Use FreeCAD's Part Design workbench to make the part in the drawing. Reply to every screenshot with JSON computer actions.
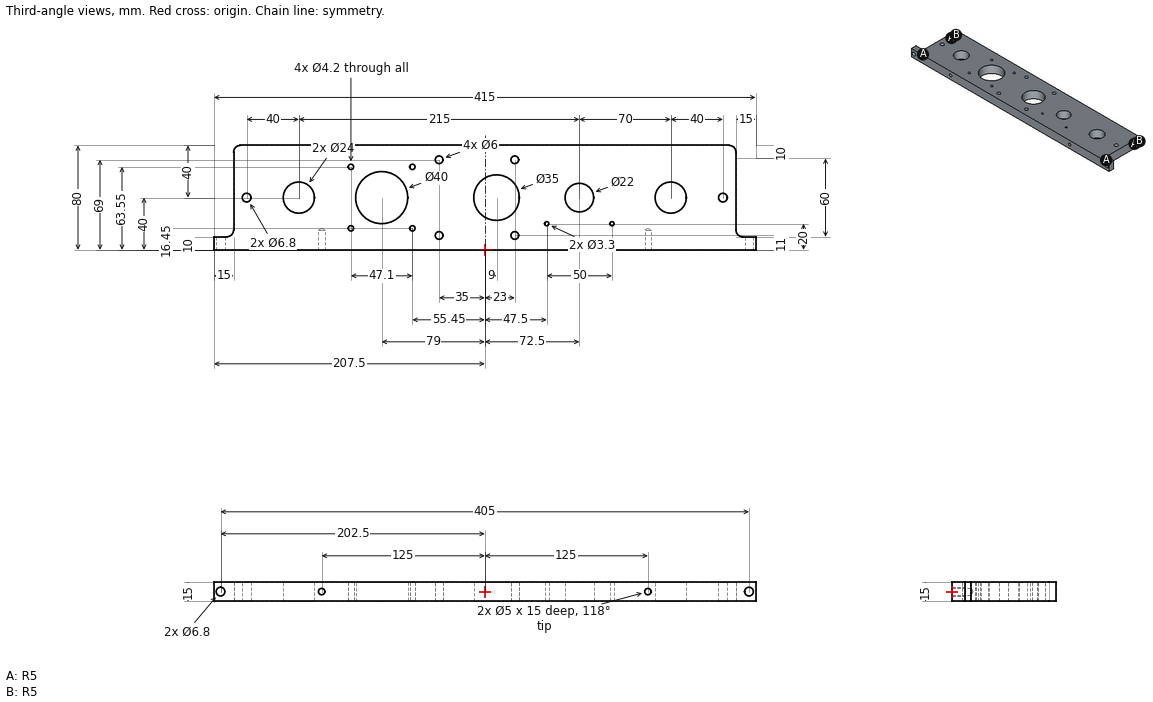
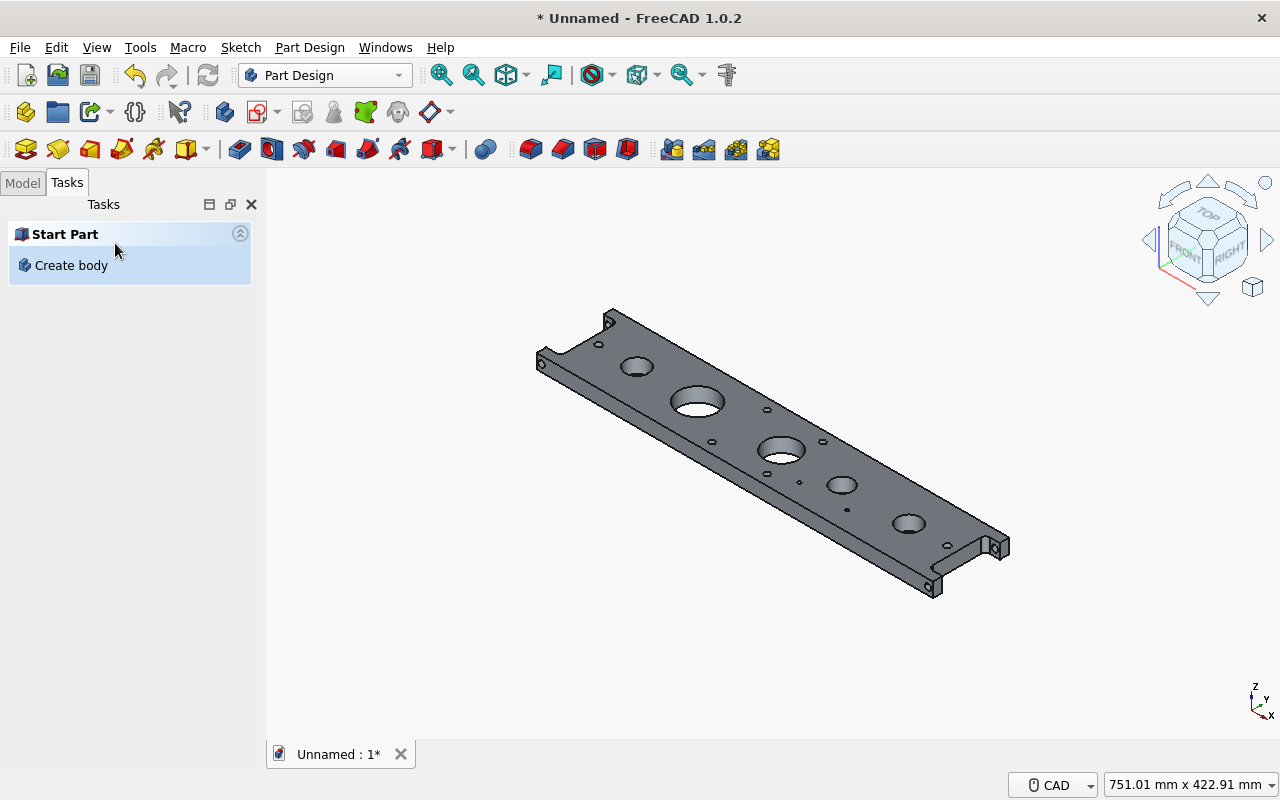
{"action": "left_click", "coordinate": [908, 497]}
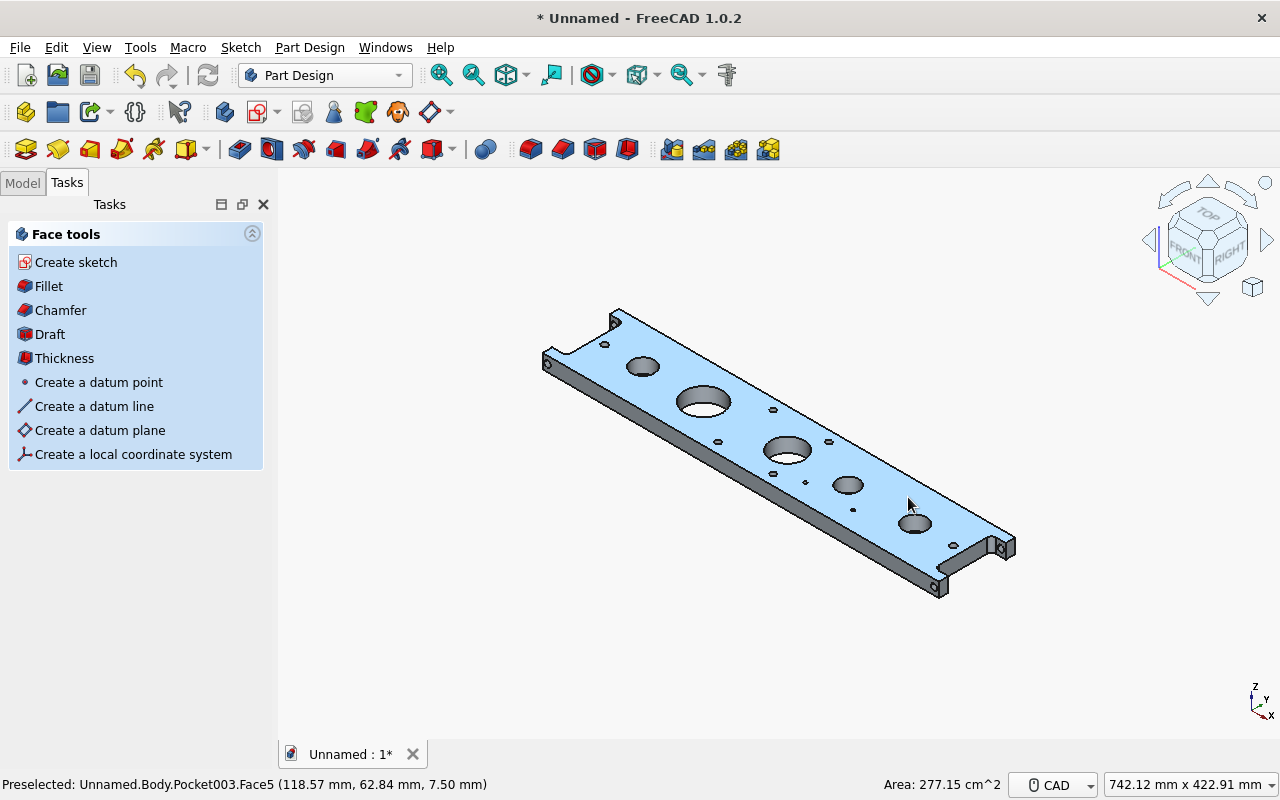
{"action": "left_click", "coordinate": [258, 112]}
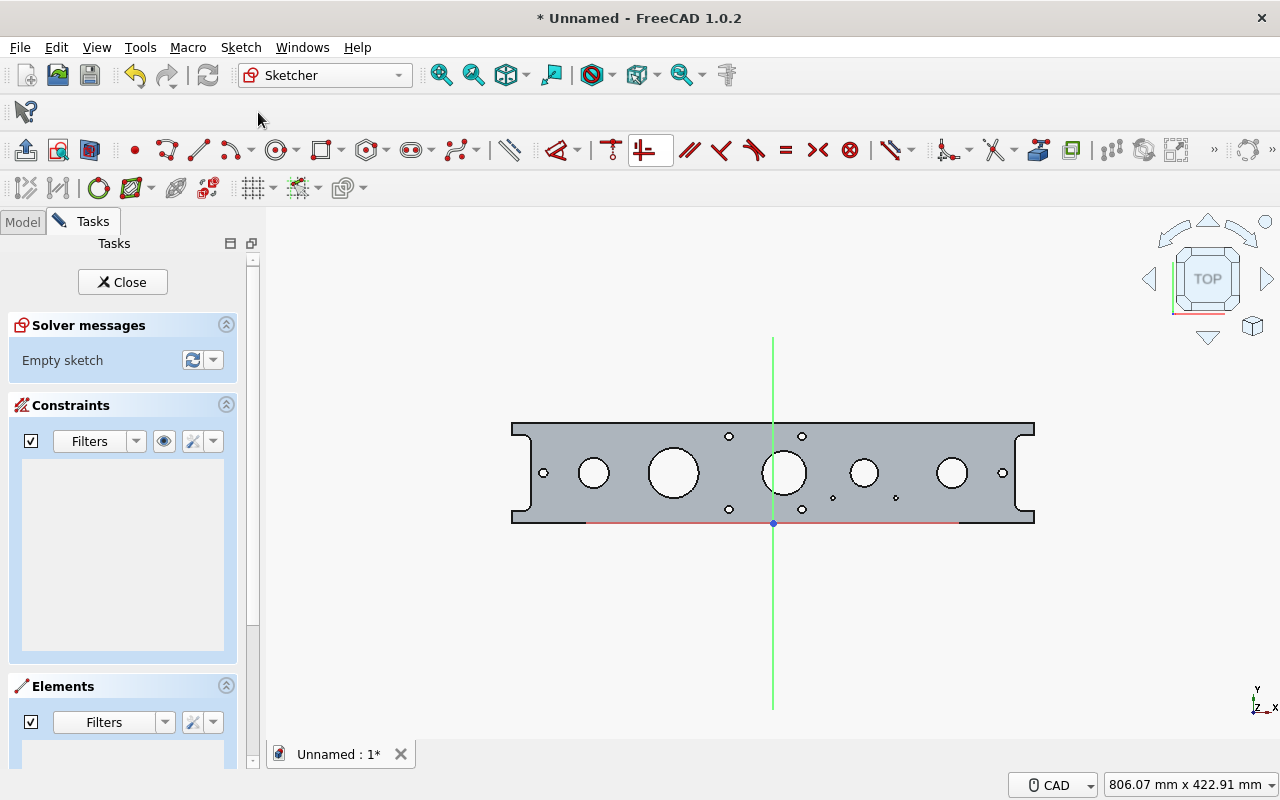
{"action": "scroll", "coordinate": [708, 485], "scroll_direction": "up", "scroll_amount": 7}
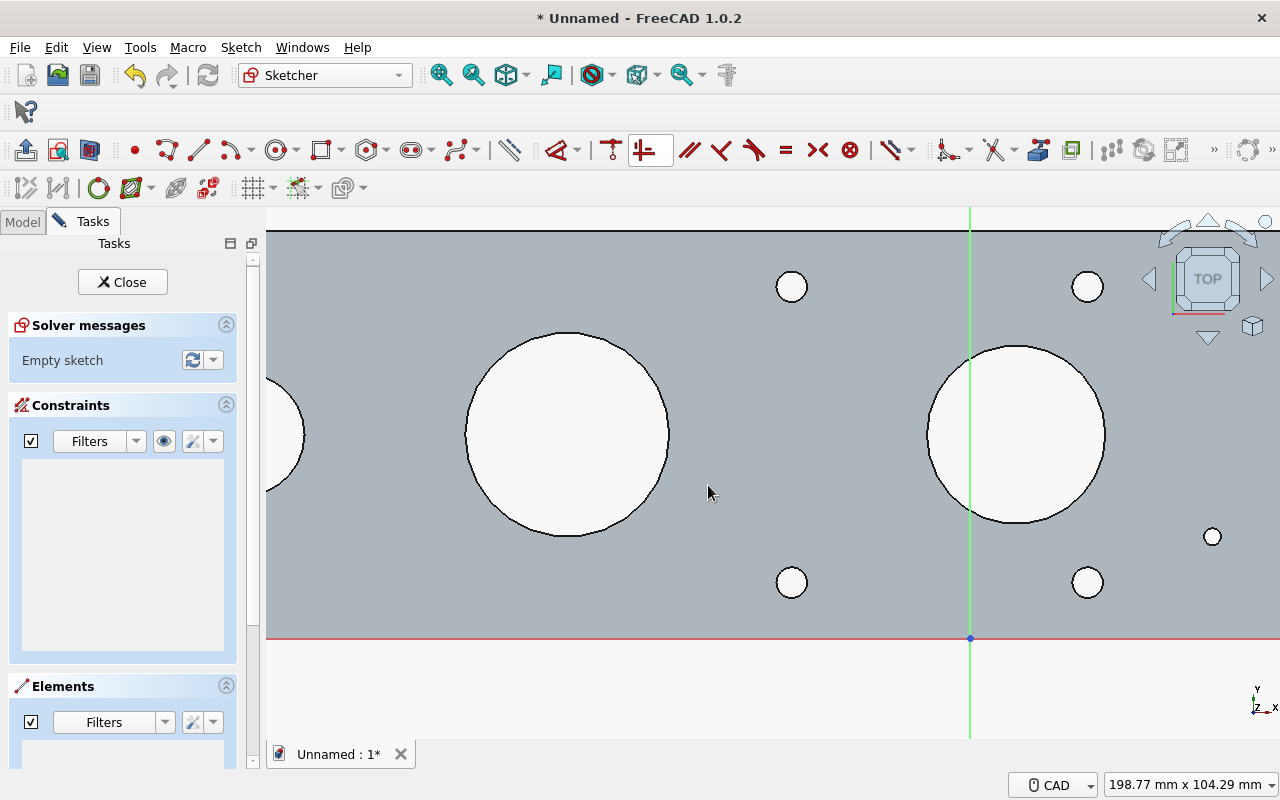
{"action": "left_click", "coordinate": [276, 150]}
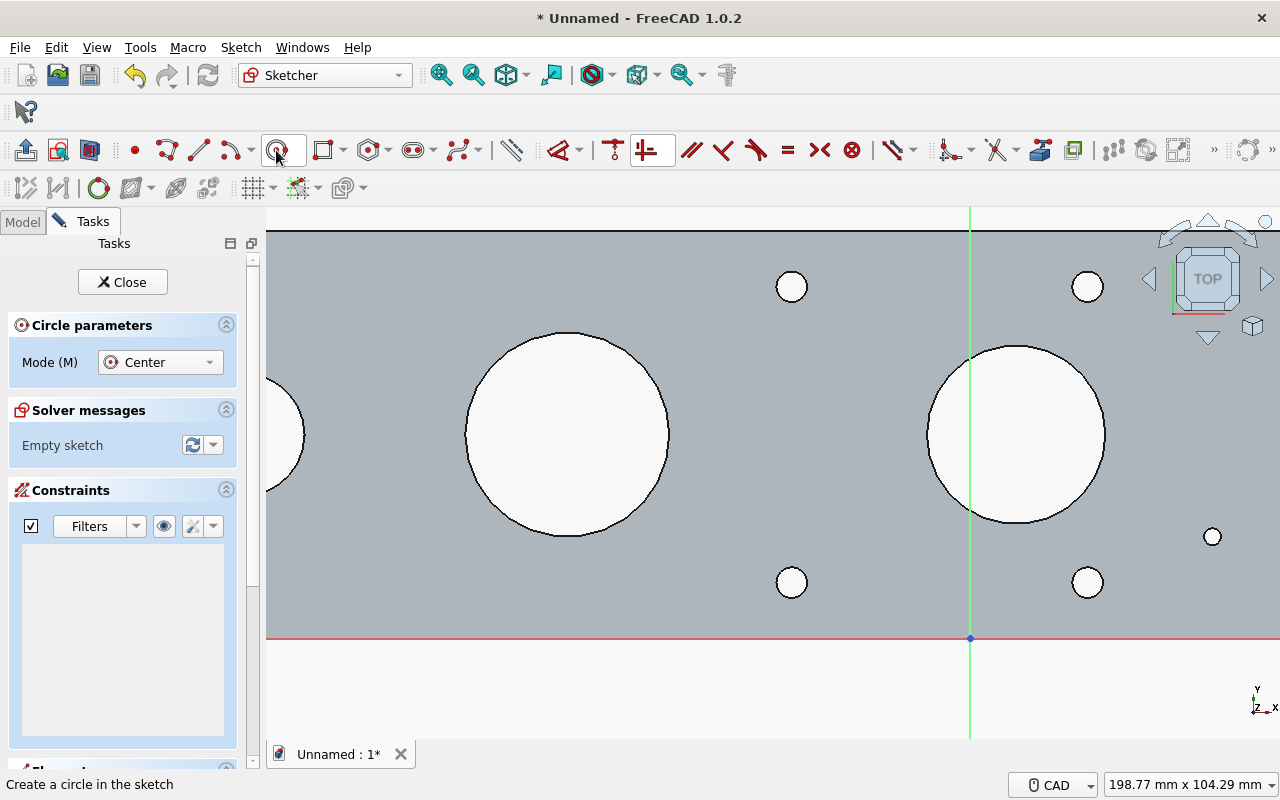
{"action": "scroll", "coordinate": [447, 315], "scroll_direction": "up", "scroll_amount": 4}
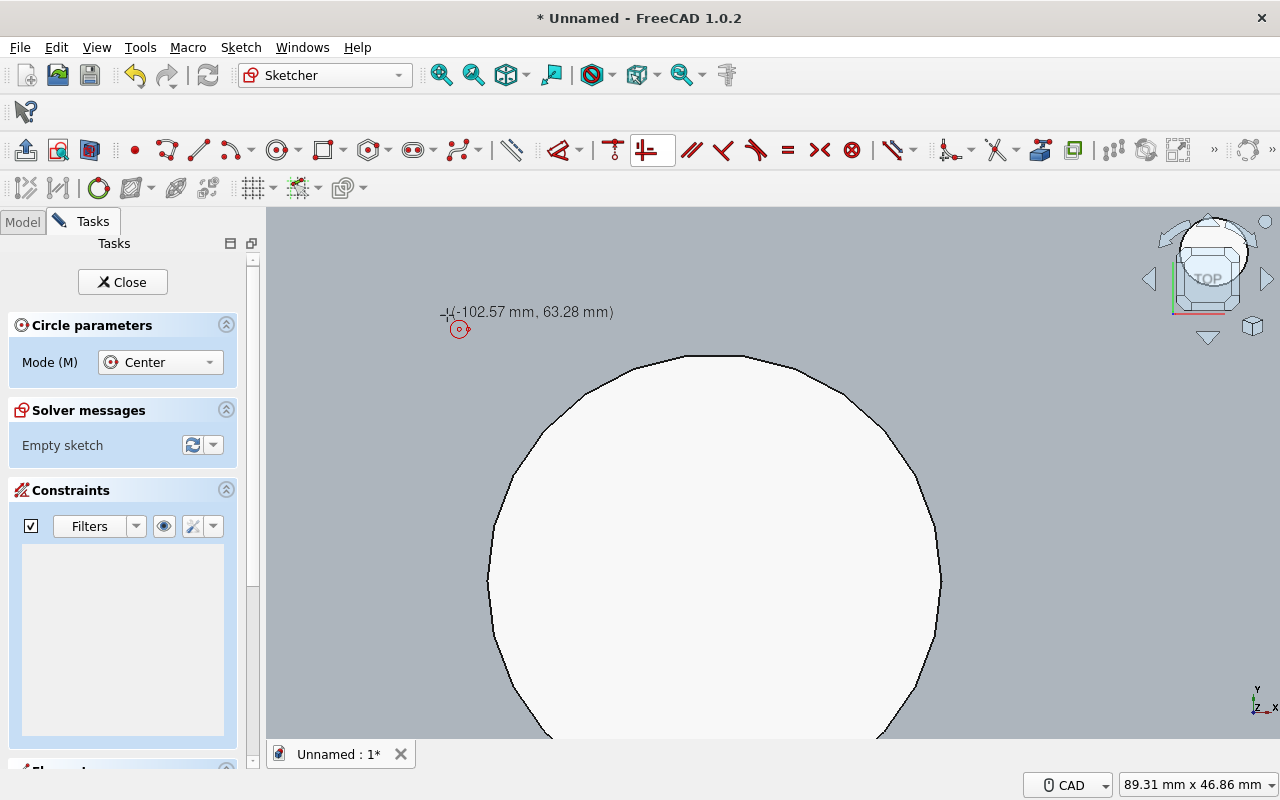
{"action": "left_click", "coordinate": [447, 314]}
{"action": "left_click", "coordinate": [464, 297]}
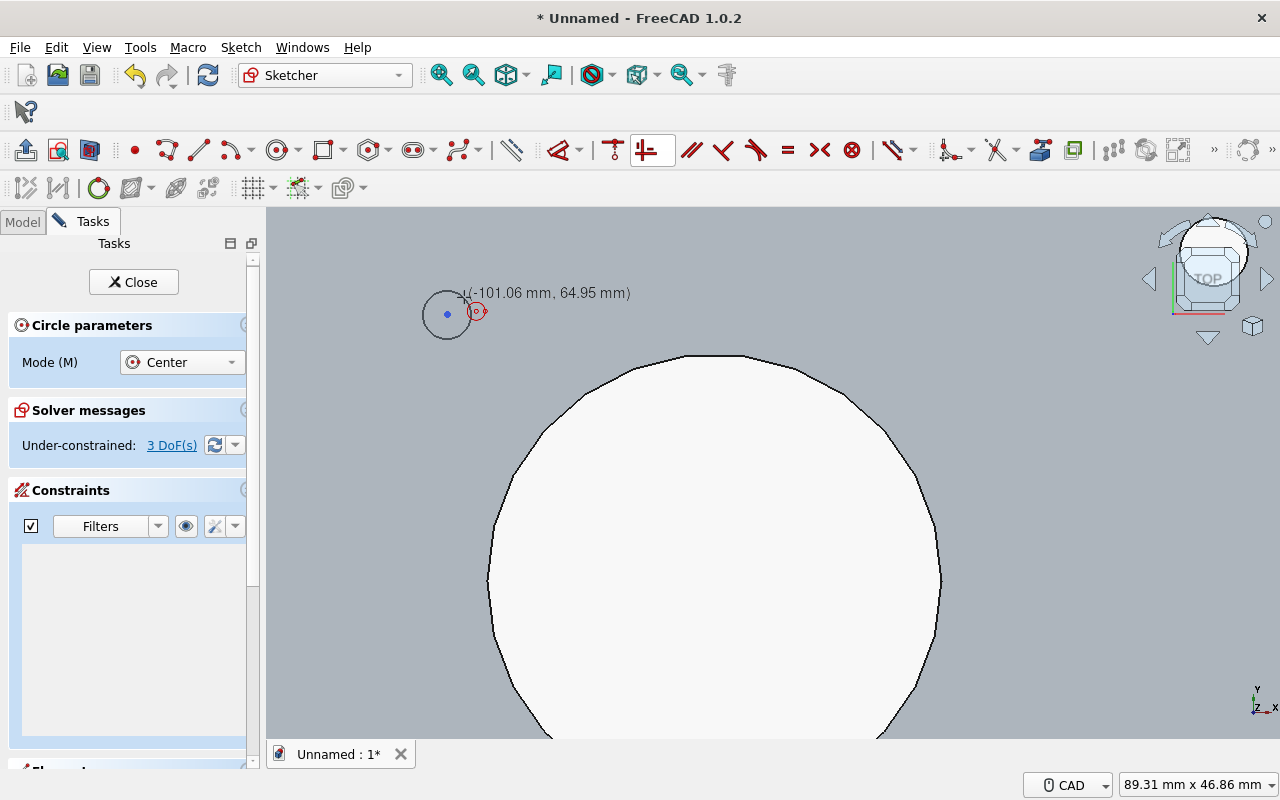
{"action": "scroll", "coordinate": [449, 318], "scroll_direction": "down", "scroll_amount": 4}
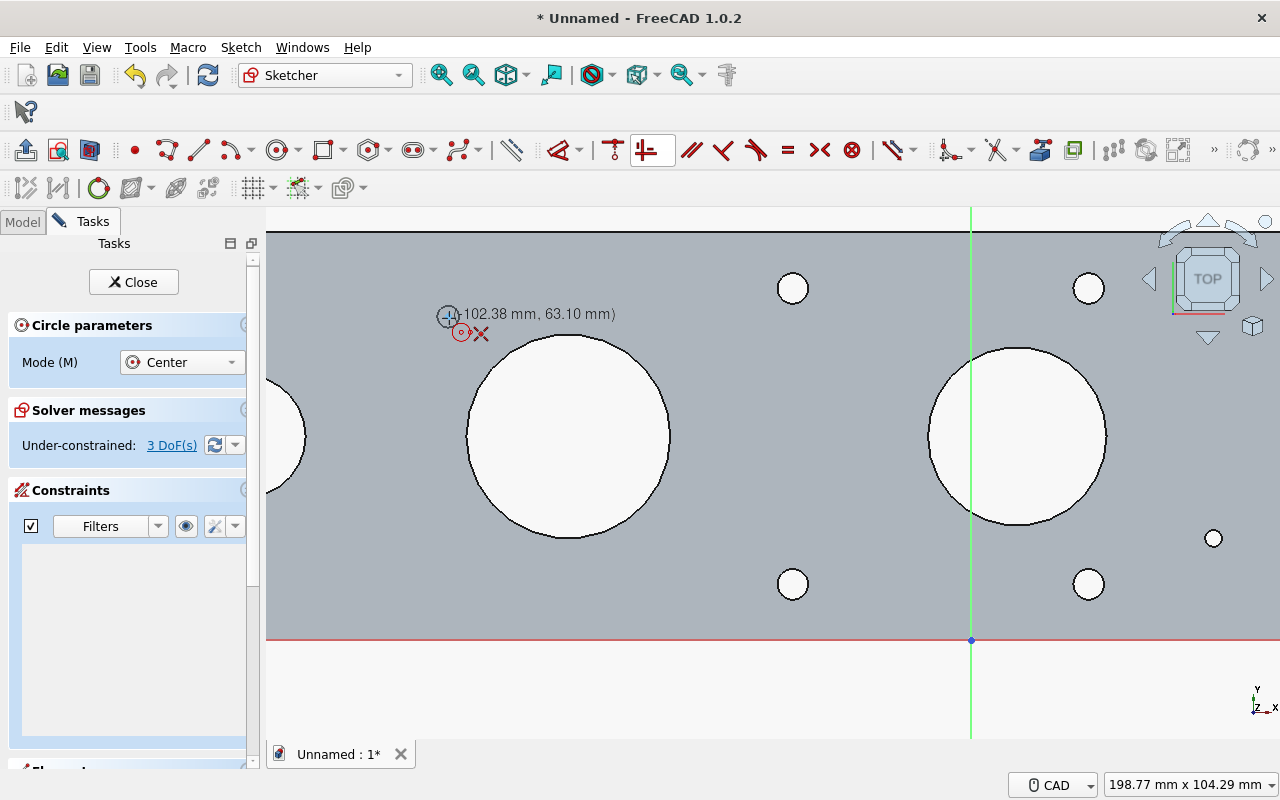
{"action": "scroll", "coordinate": [688, 557], "scroll_direction": "up", "scroll_amount": 4}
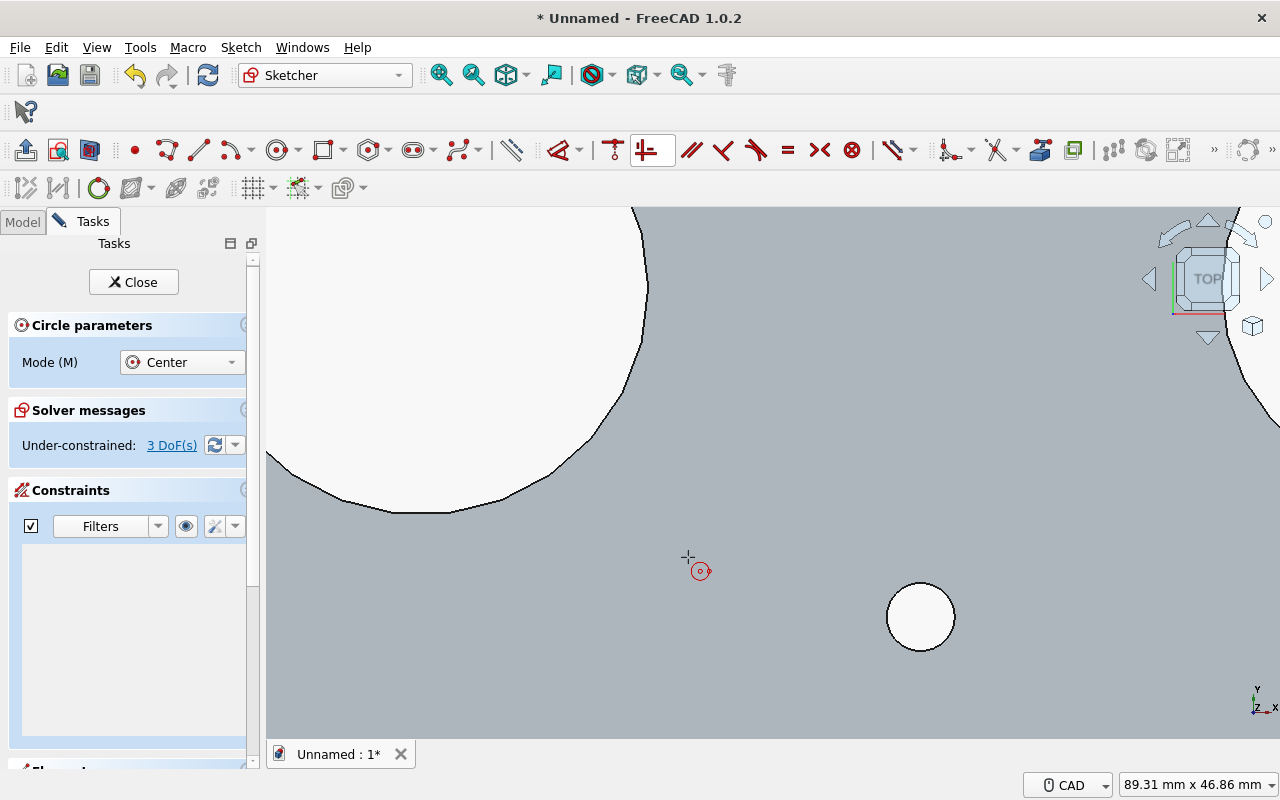
{"action": "left_click", "coordinate": [689, 555]}
{"action": "left_click", "coordinate": [705, 538]}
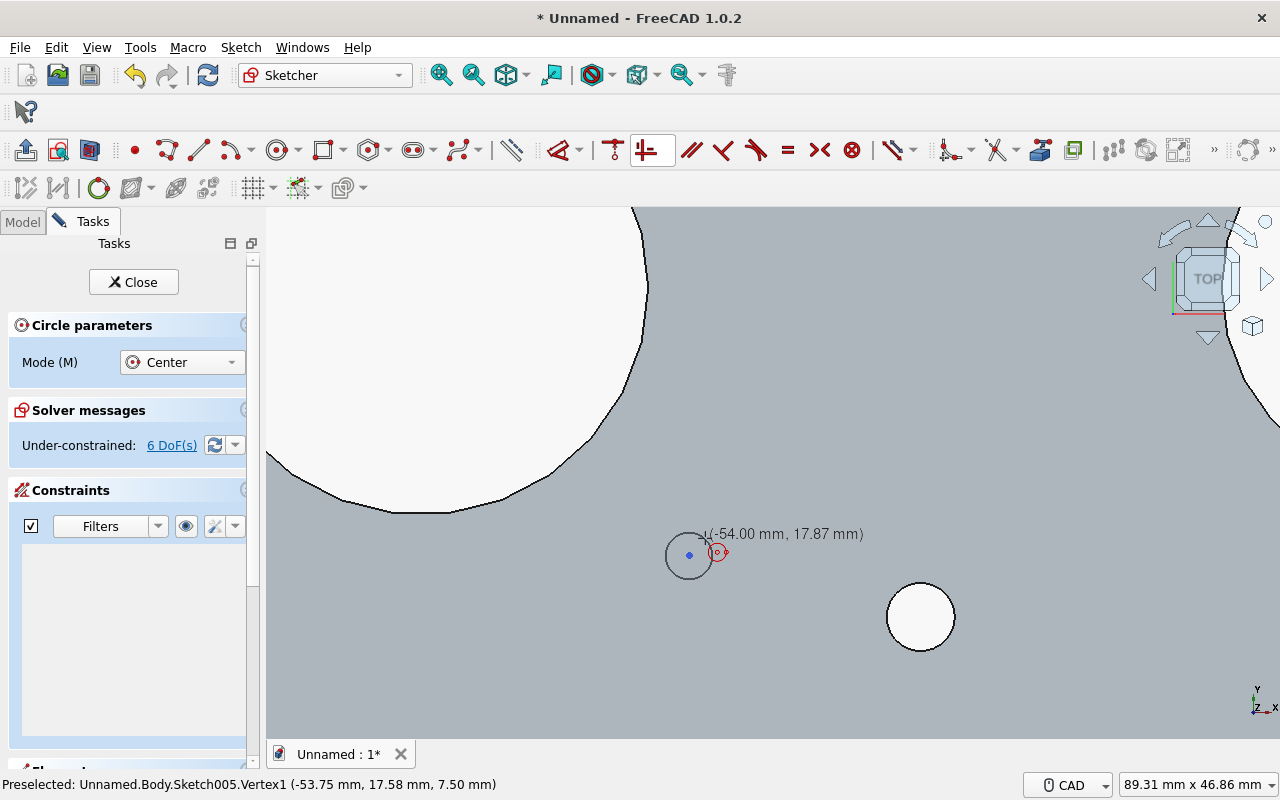
{"action": "scroll", "coordinate": [689, 558], "scroll_direction": "down", "scroll_amount": 4}